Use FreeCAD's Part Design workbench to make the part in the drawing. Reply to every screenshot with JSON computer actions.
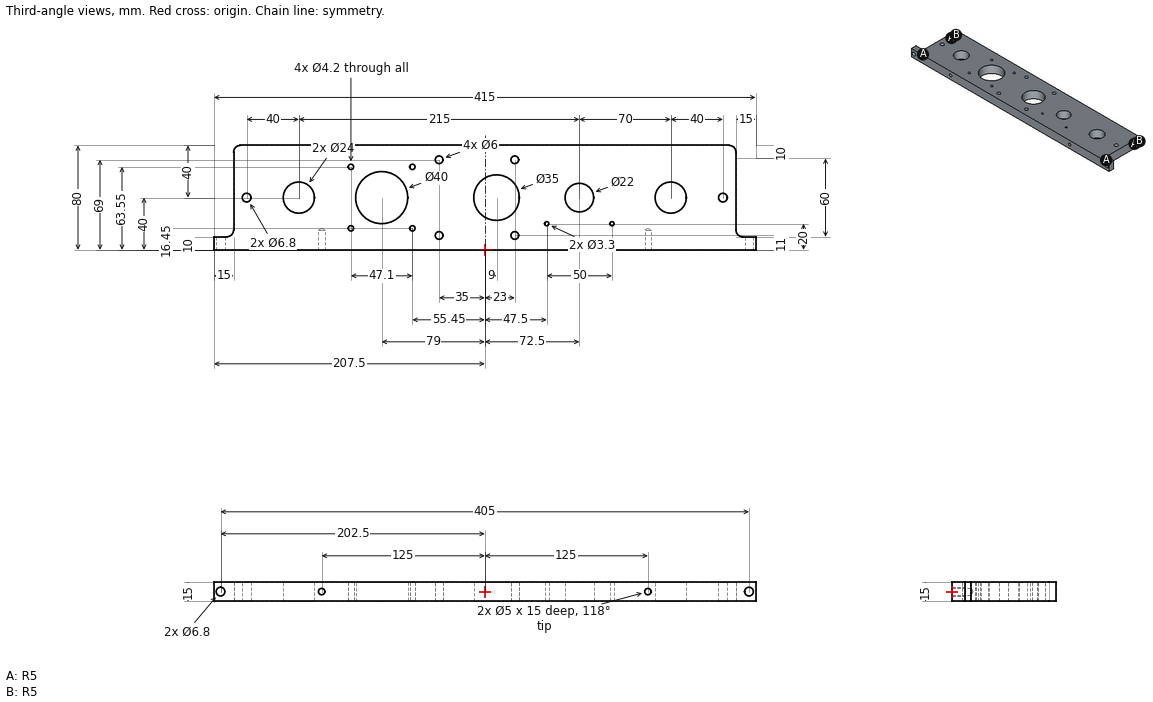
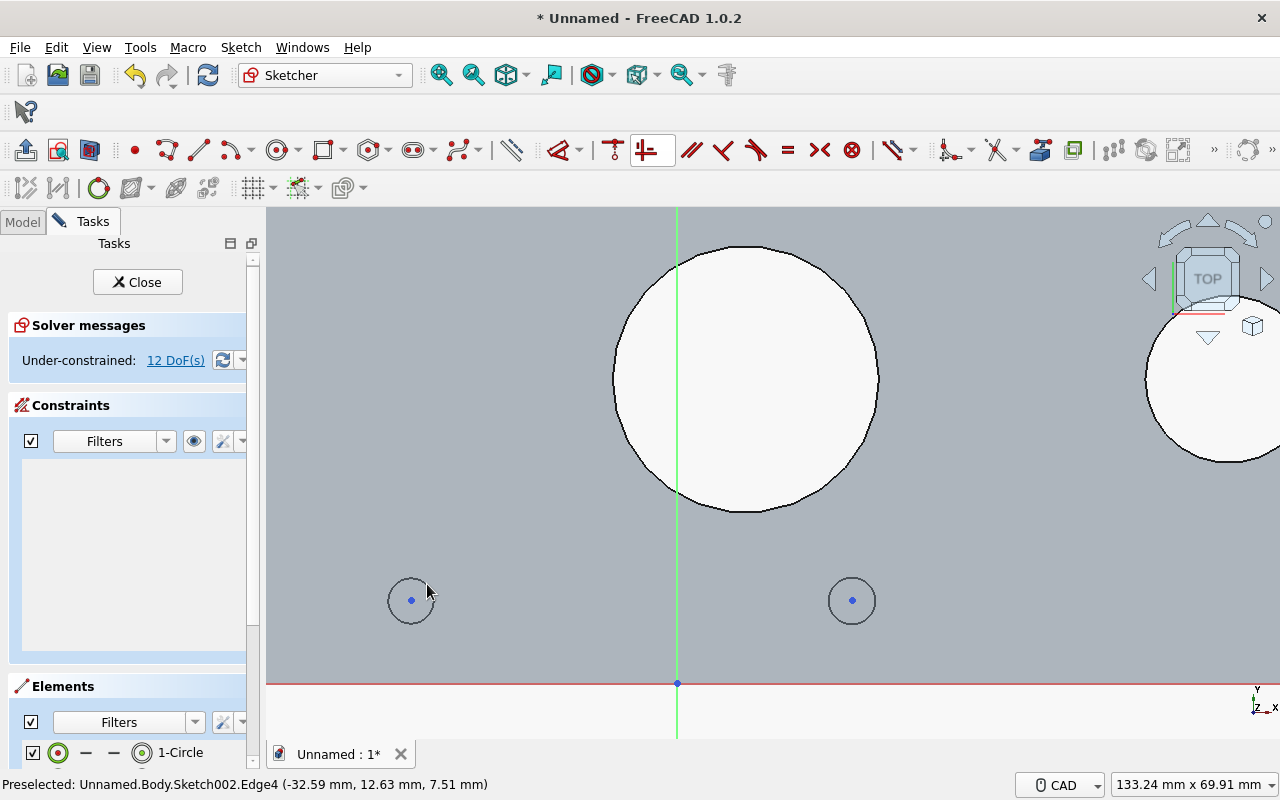
{"action": "scroll", "coordinate": [853, 601], "scroll_direction": "down", "scroll_amount": 2}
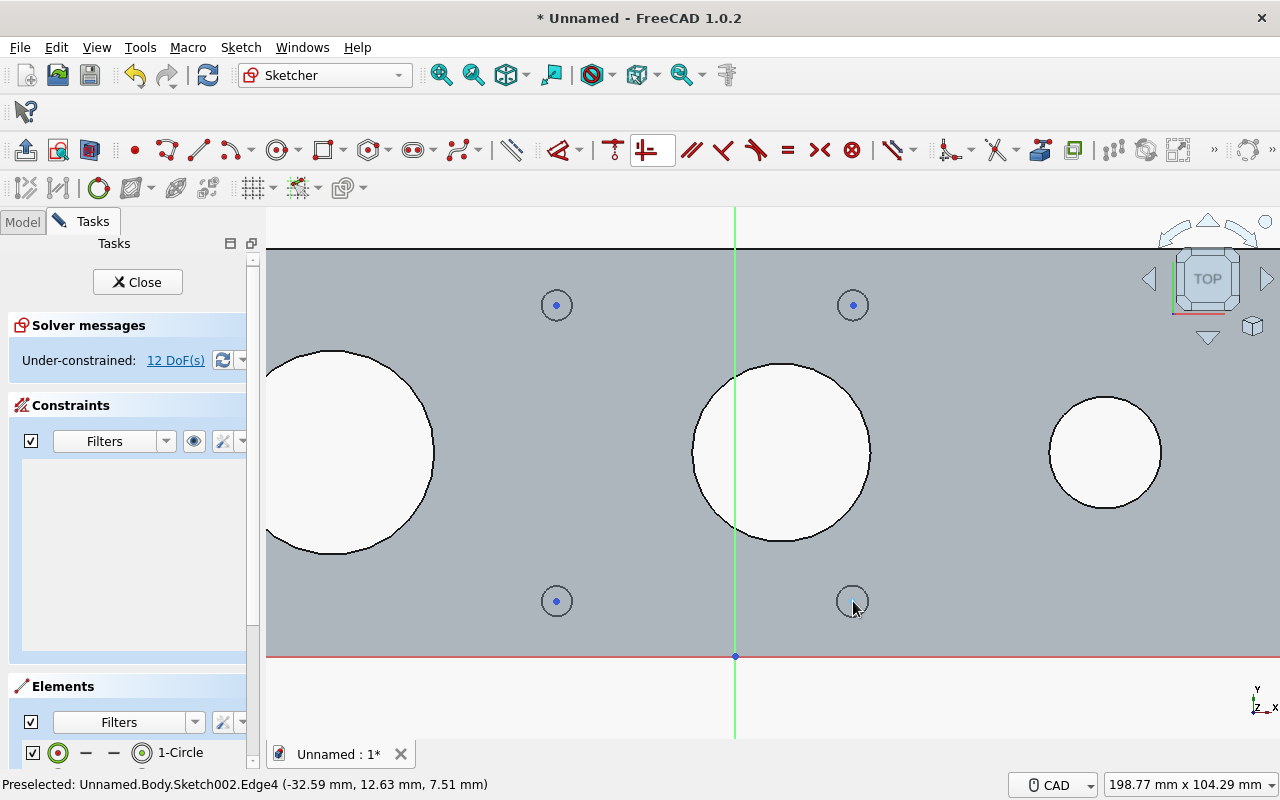
{"action": "left_click", "coordinate": [567, 295]}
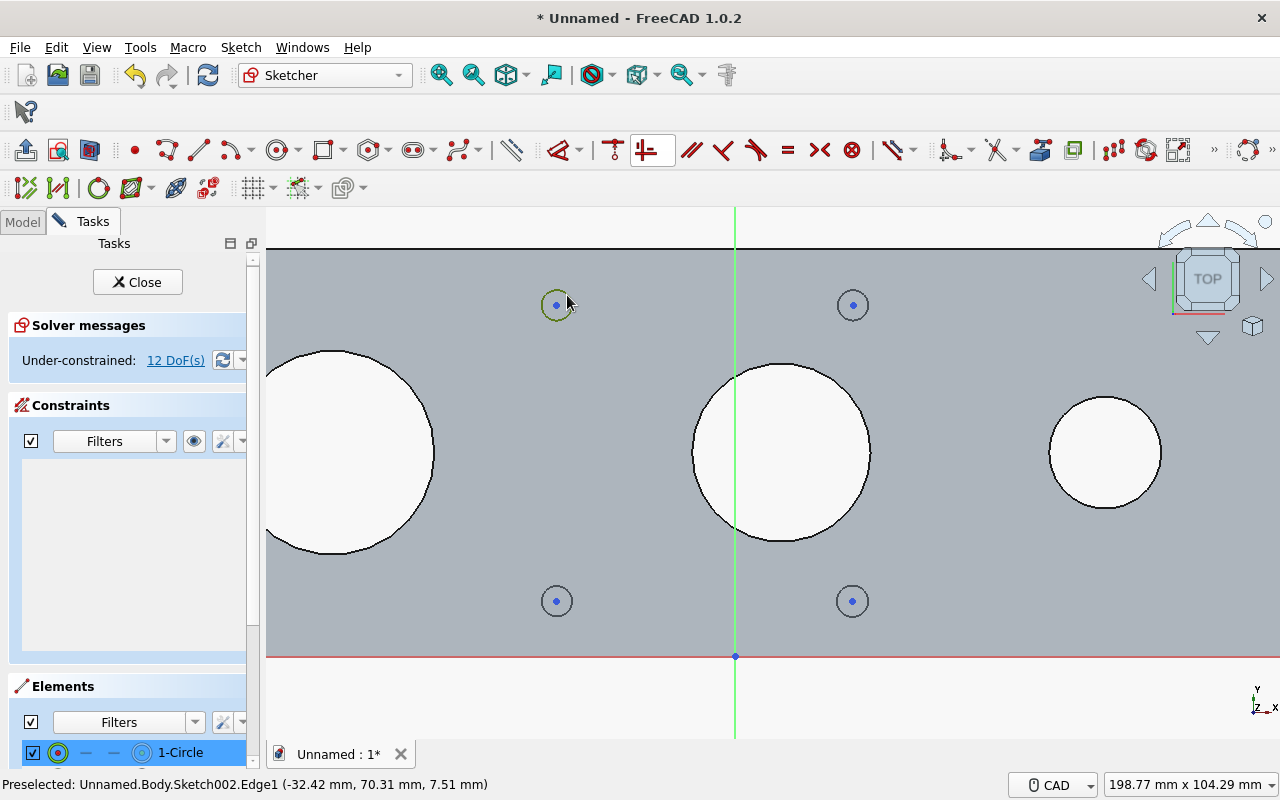
{"action": "left_click", "coordinate": [864, 295]}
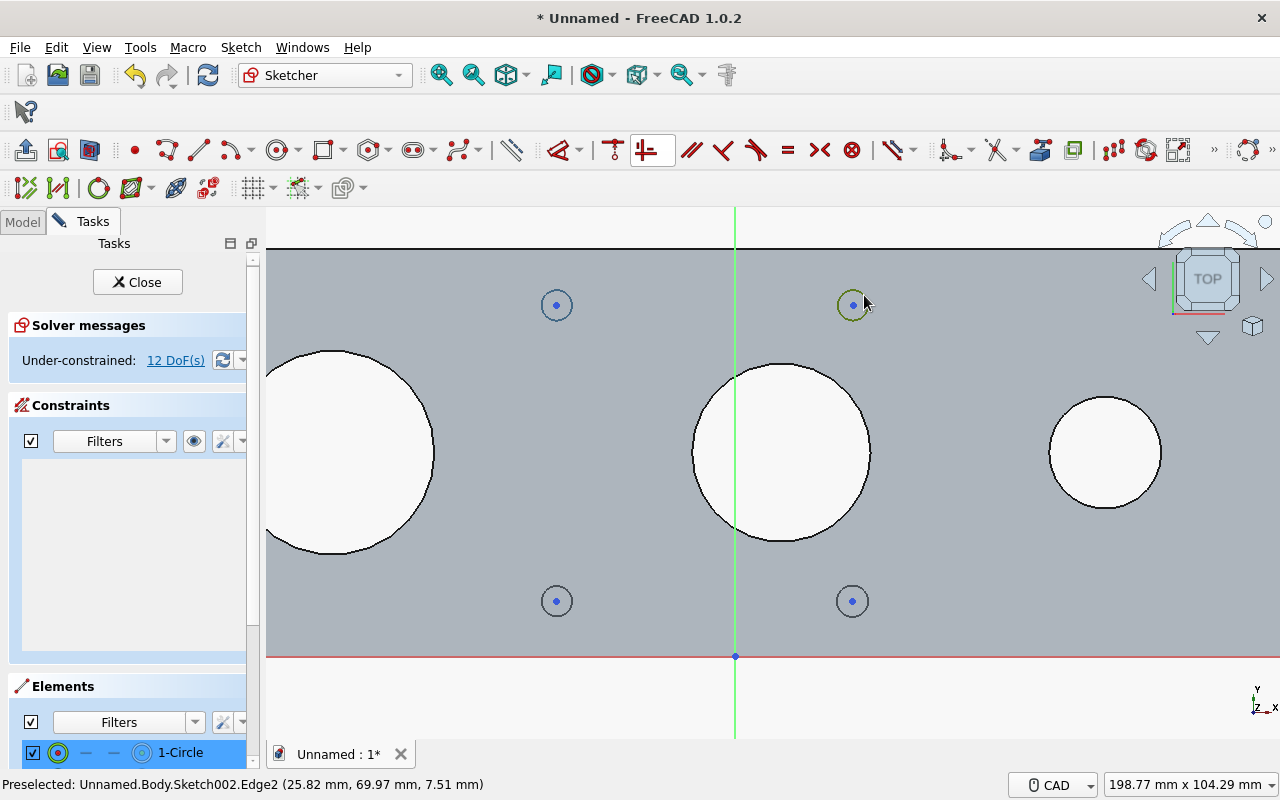
{"action": "left_click", "coordinate": [864, 590]}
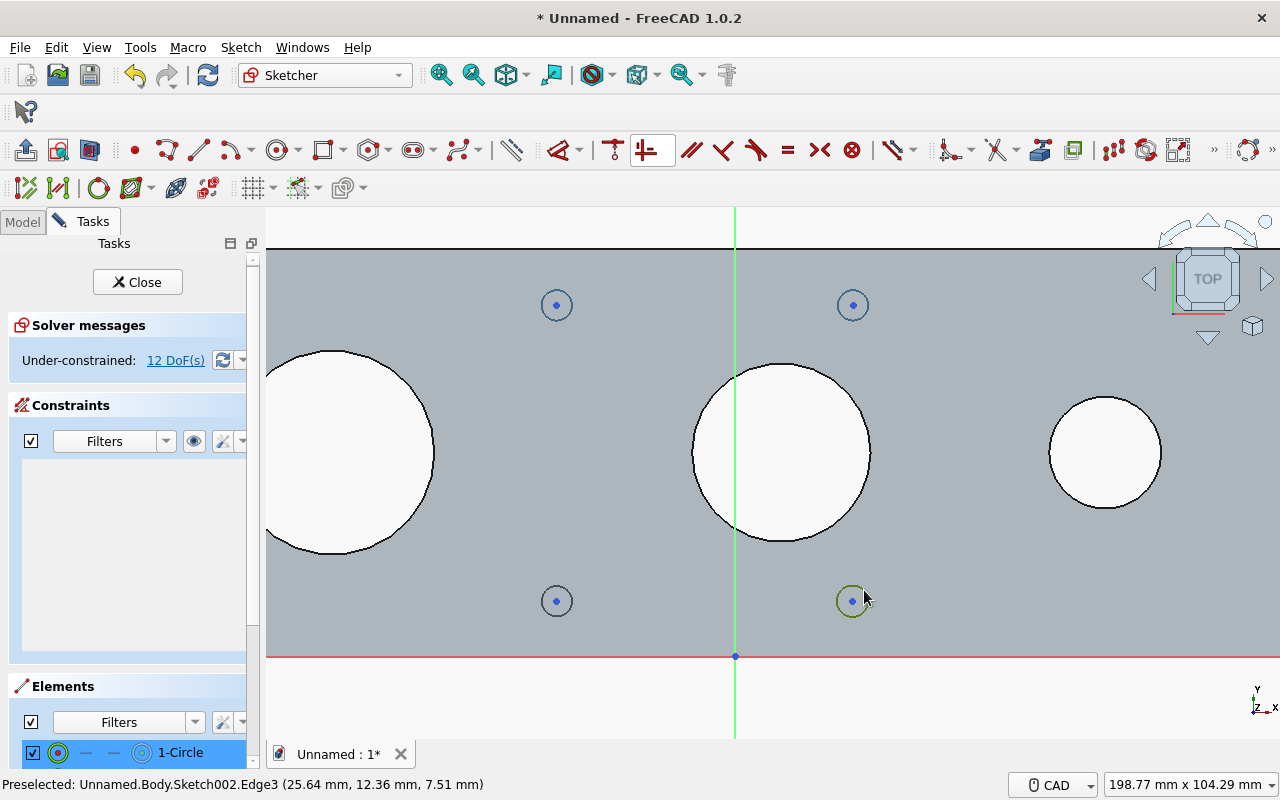
{"action": "left_click", "coordinate": [568, 590]}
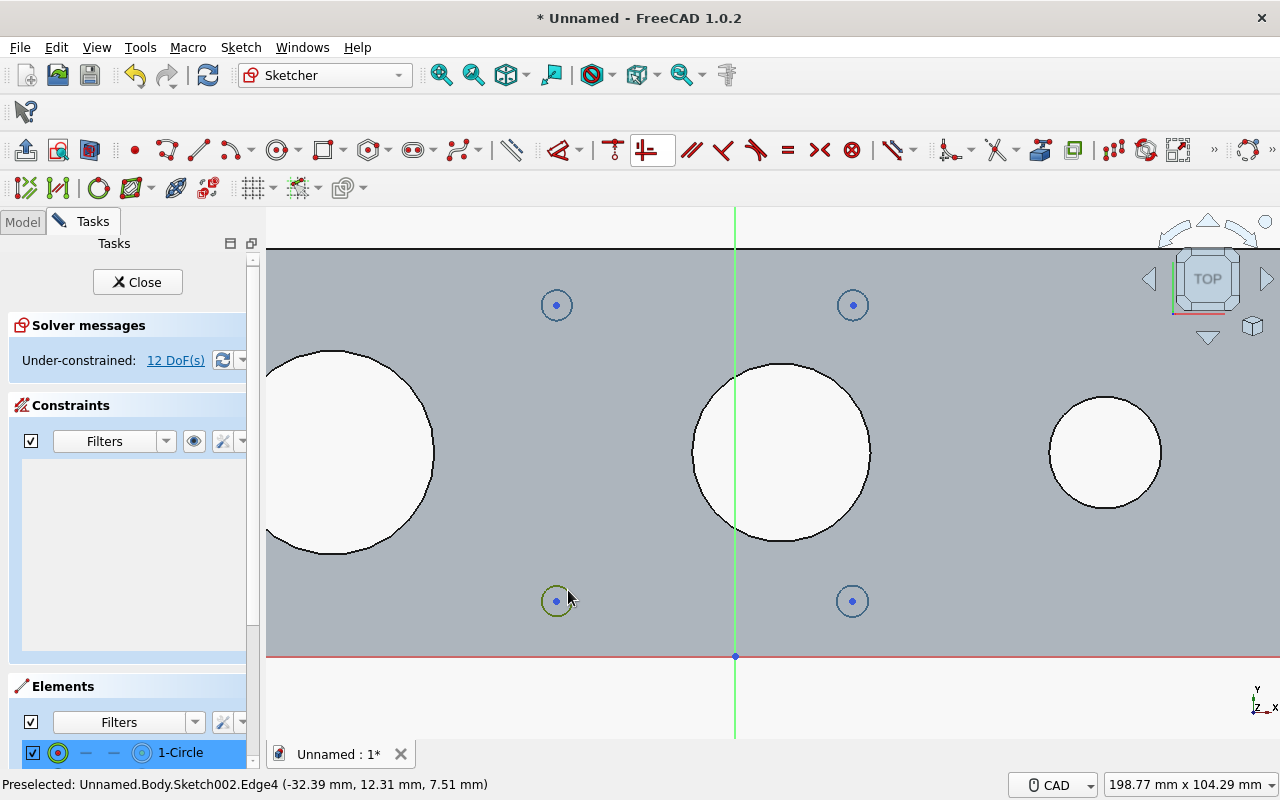
{"action": "left_click", "coordinate": [788, 150]}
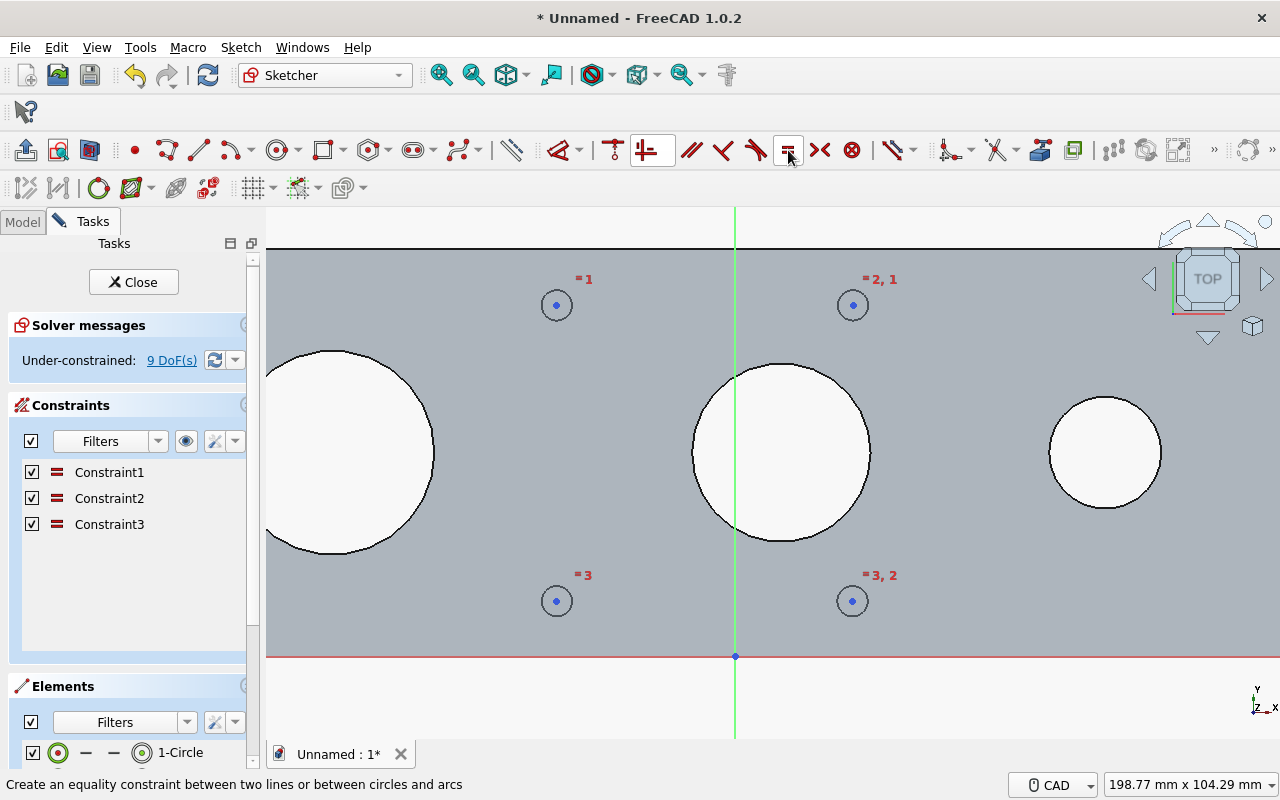
{"action": "left_click", "coordinate": [557, 305]}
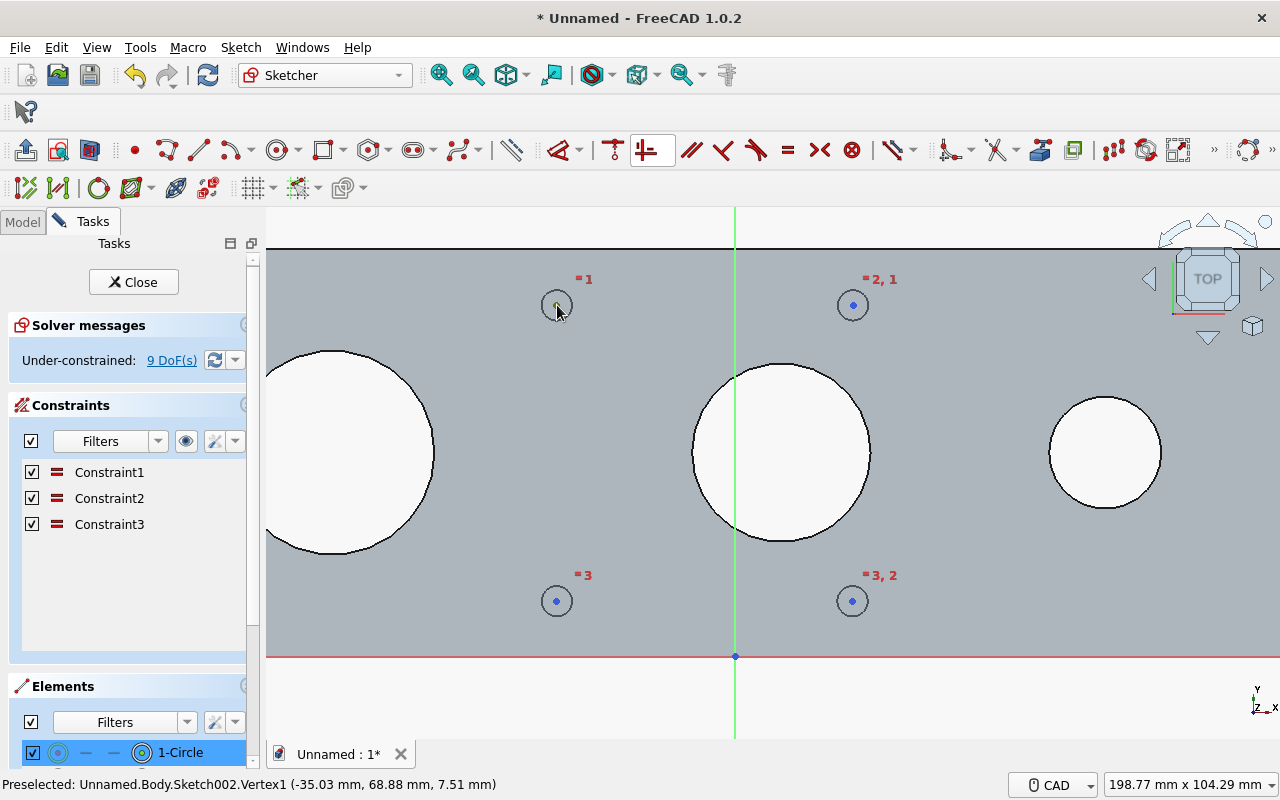
{"action": "left_click", "coordinate": [853, 305]}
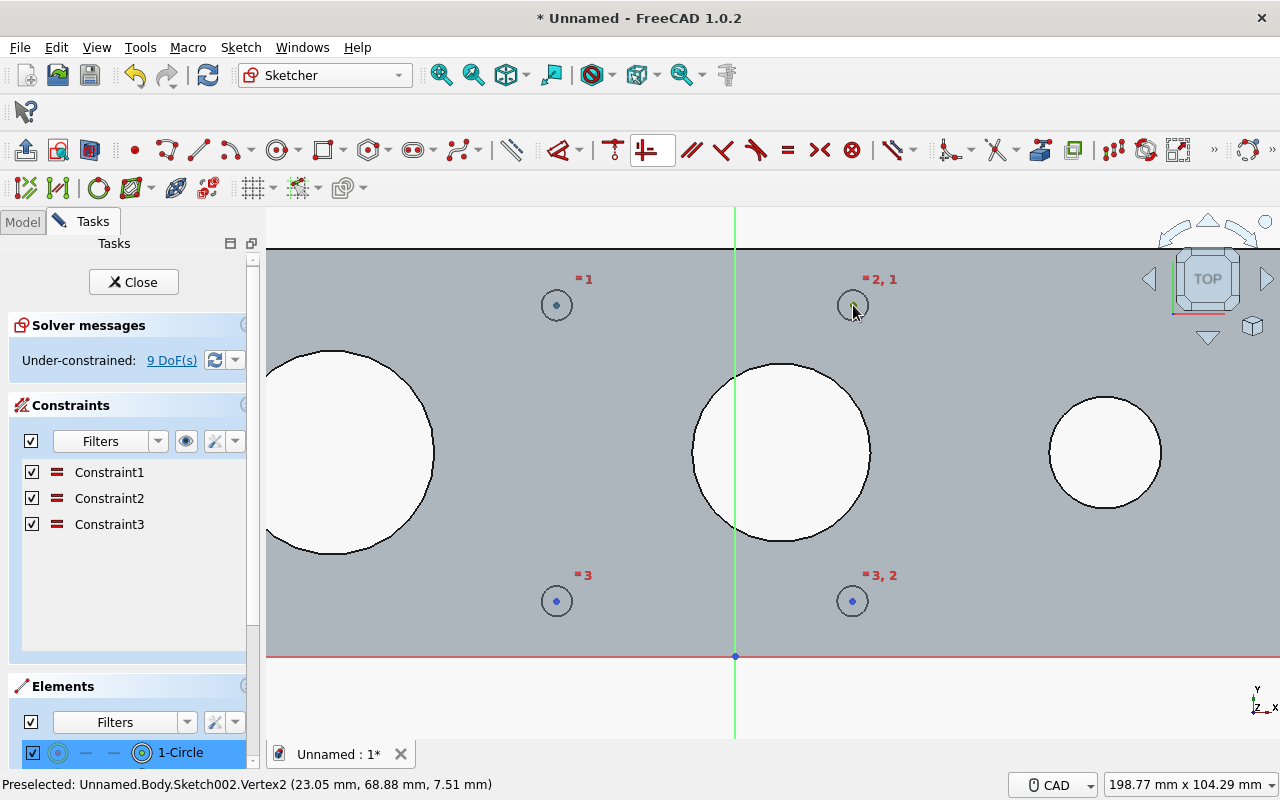
{"action": "key", "text": "h"}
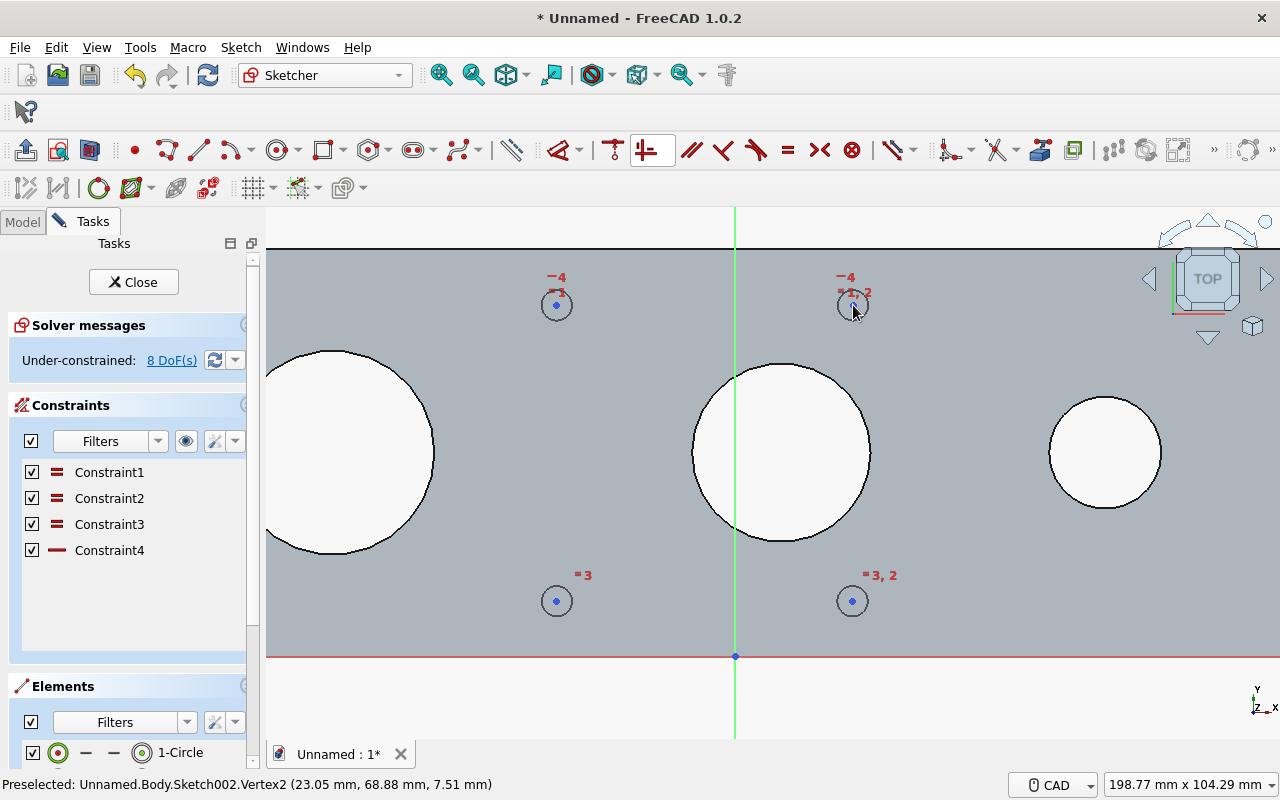
{"action": "left_click", "coordinate": [853, 305]}